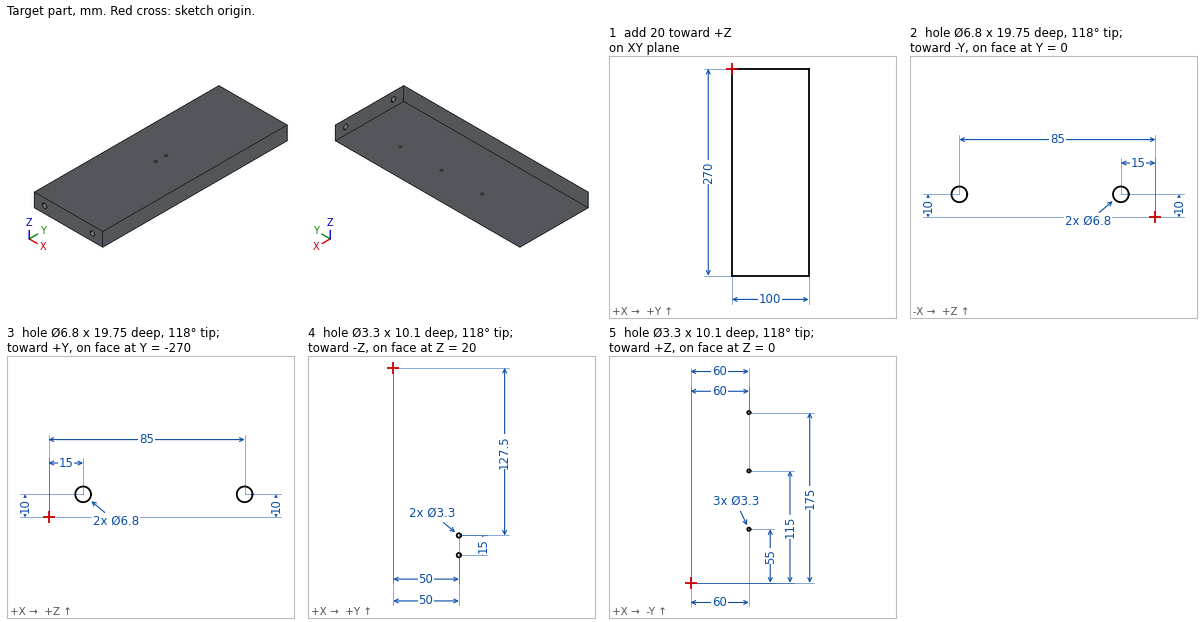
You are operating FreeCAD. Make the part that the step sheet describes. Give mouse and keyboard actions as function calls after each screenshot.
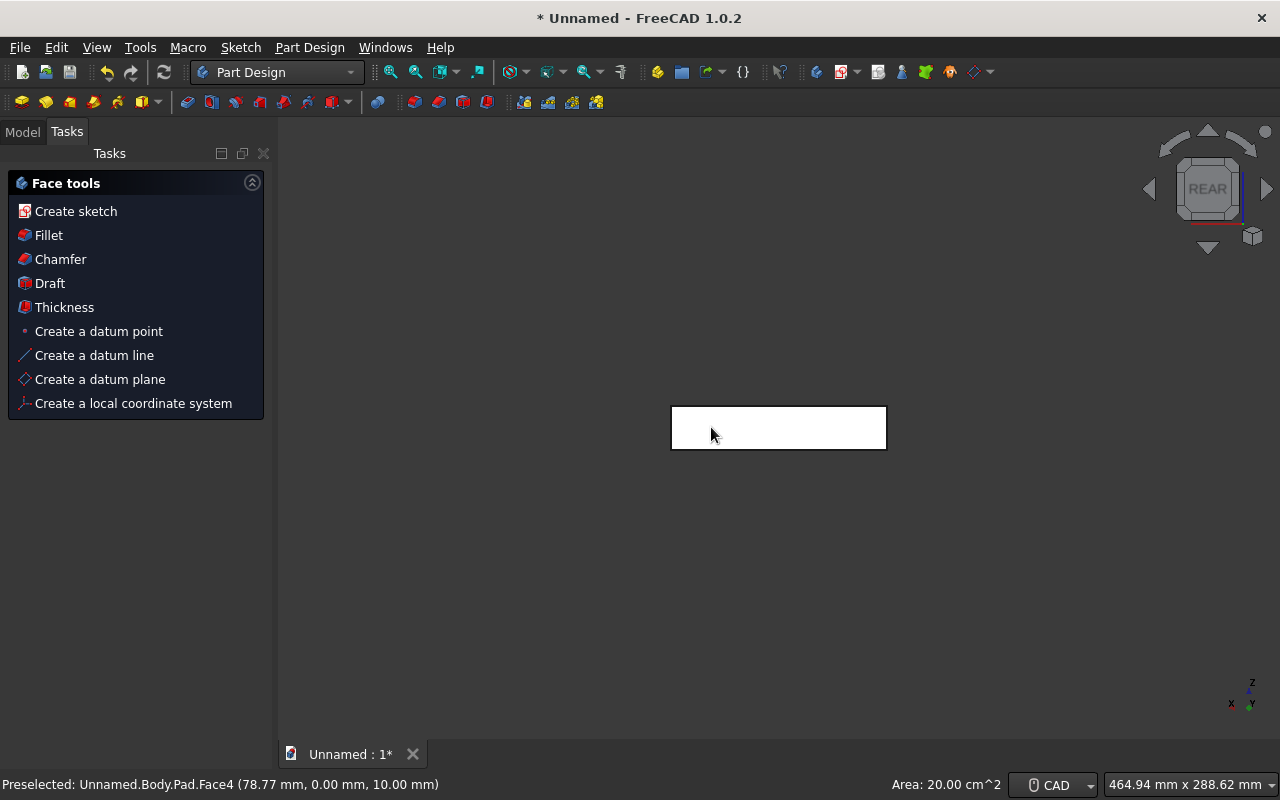
click(842, 72)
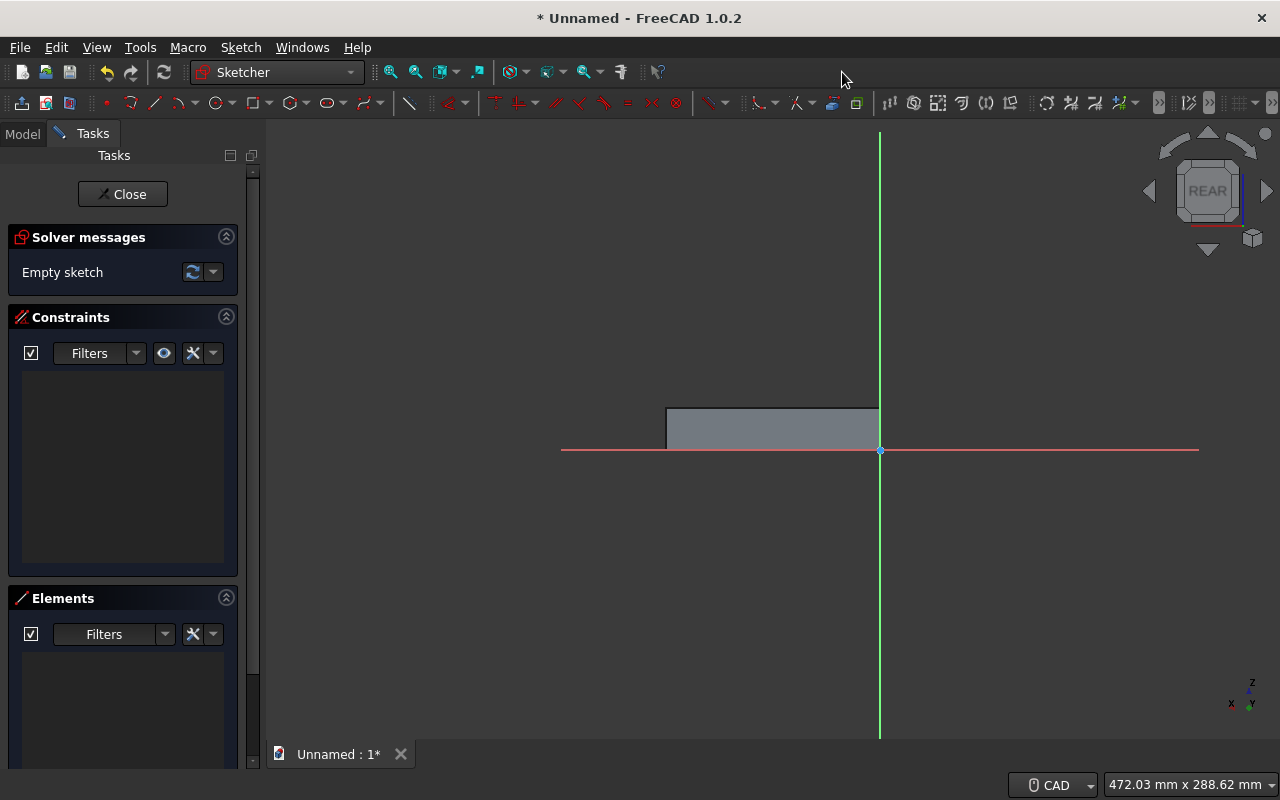
scroll(820, 439, up, 6)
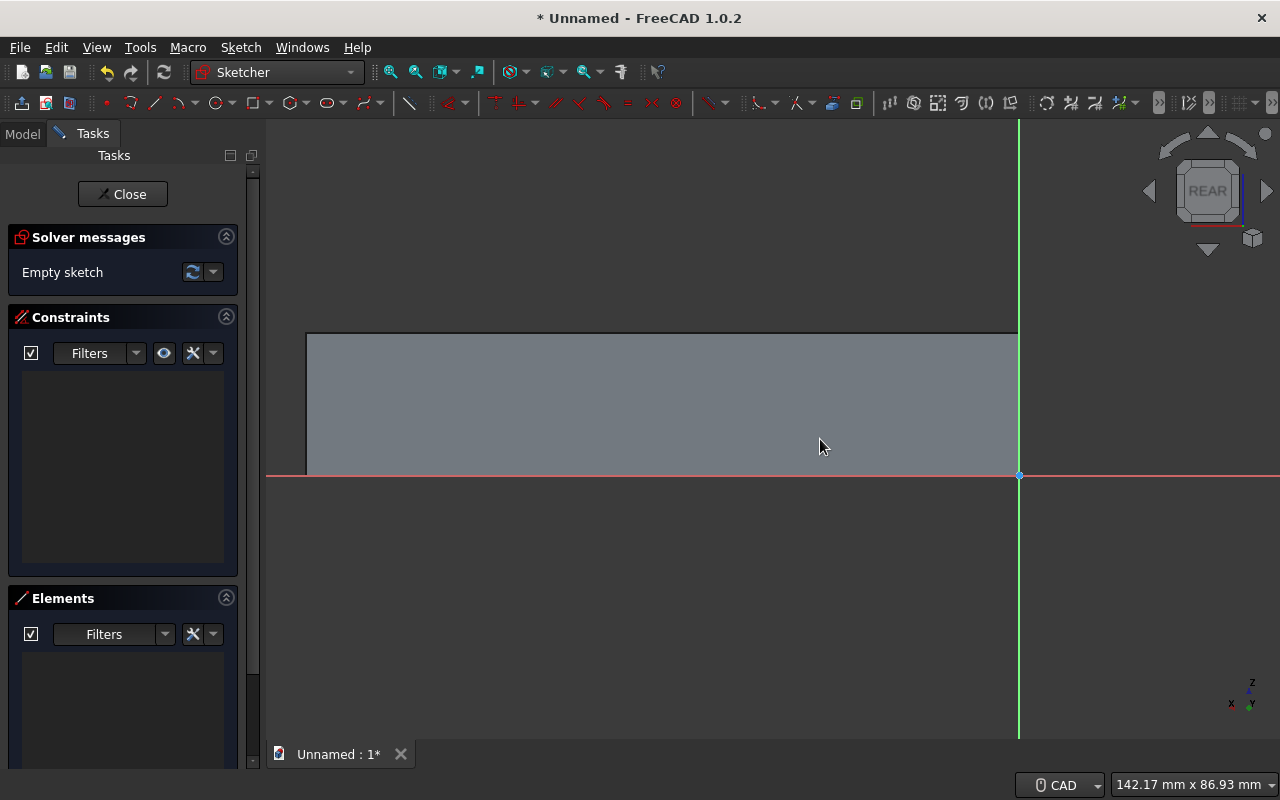
click(216, 104)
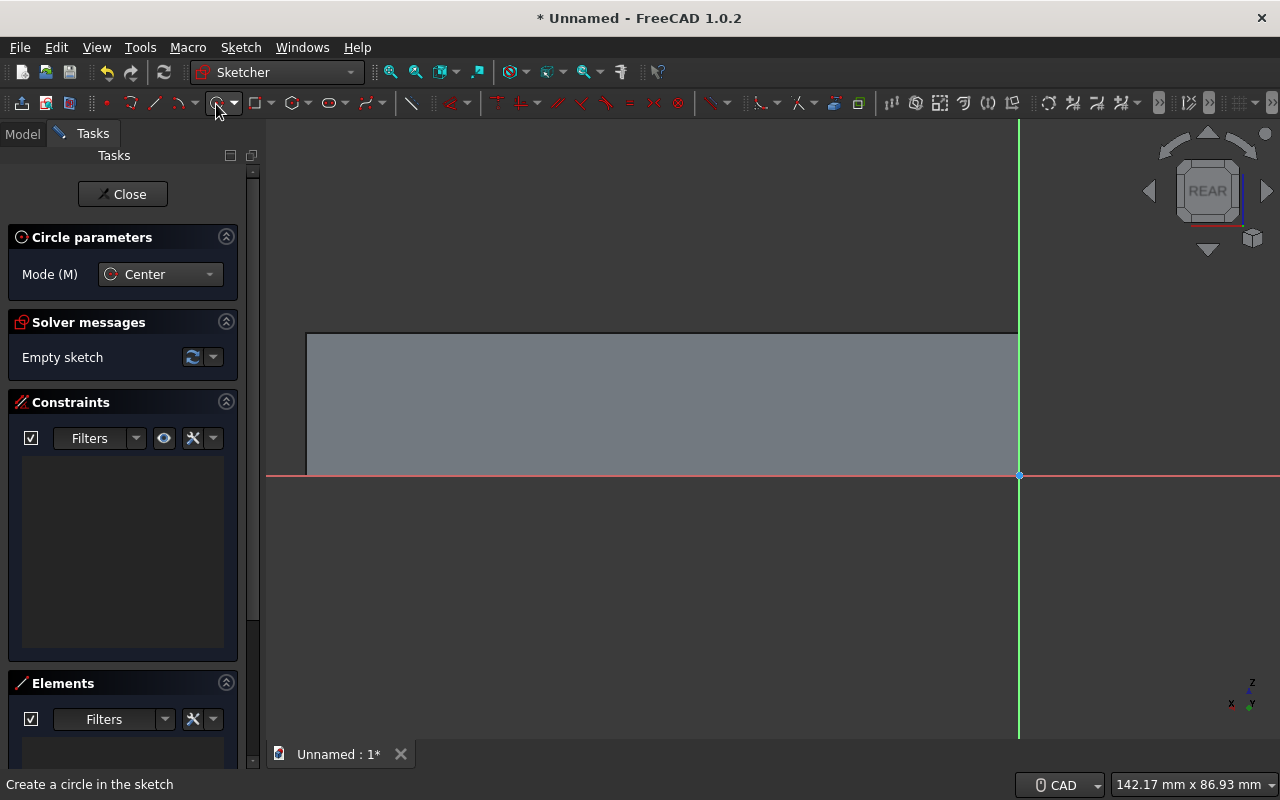
click(912, 405)
click(929, 387)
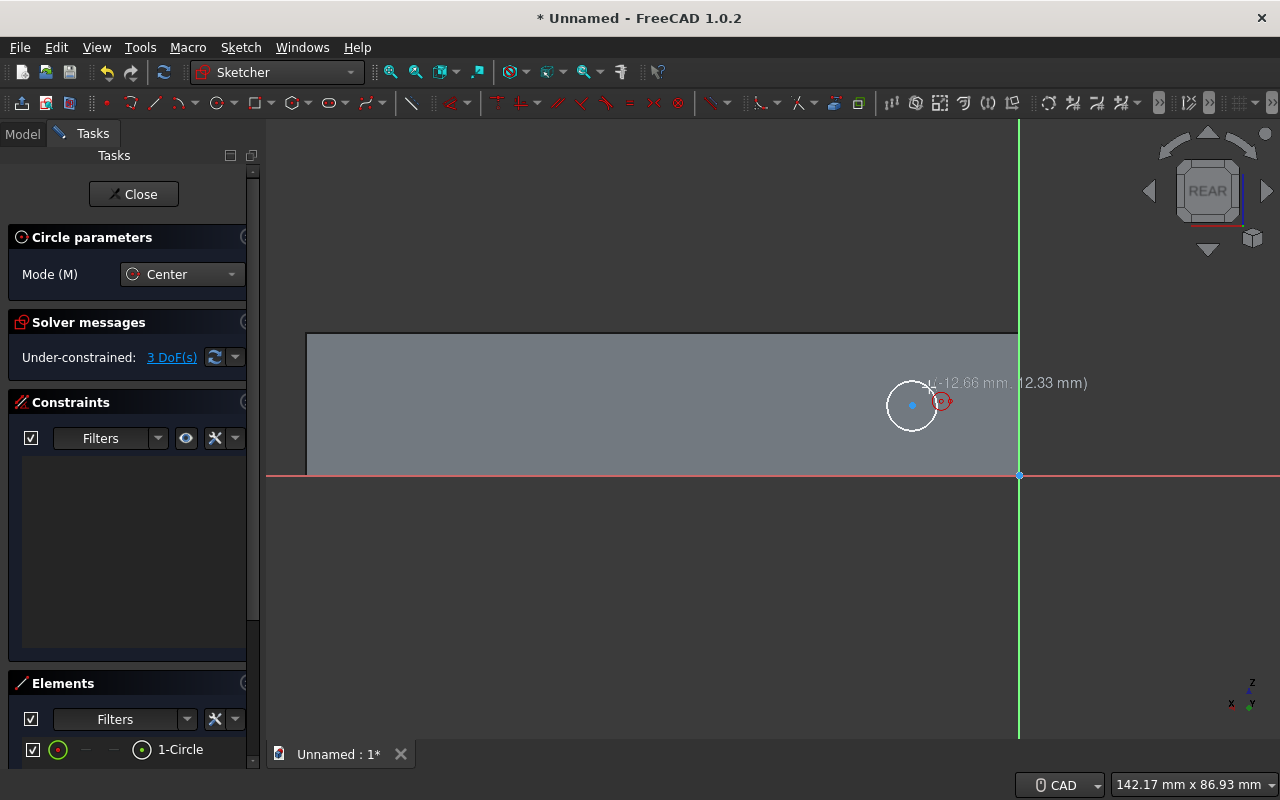
click(413, 405)
click(430, 387)
key(Escape)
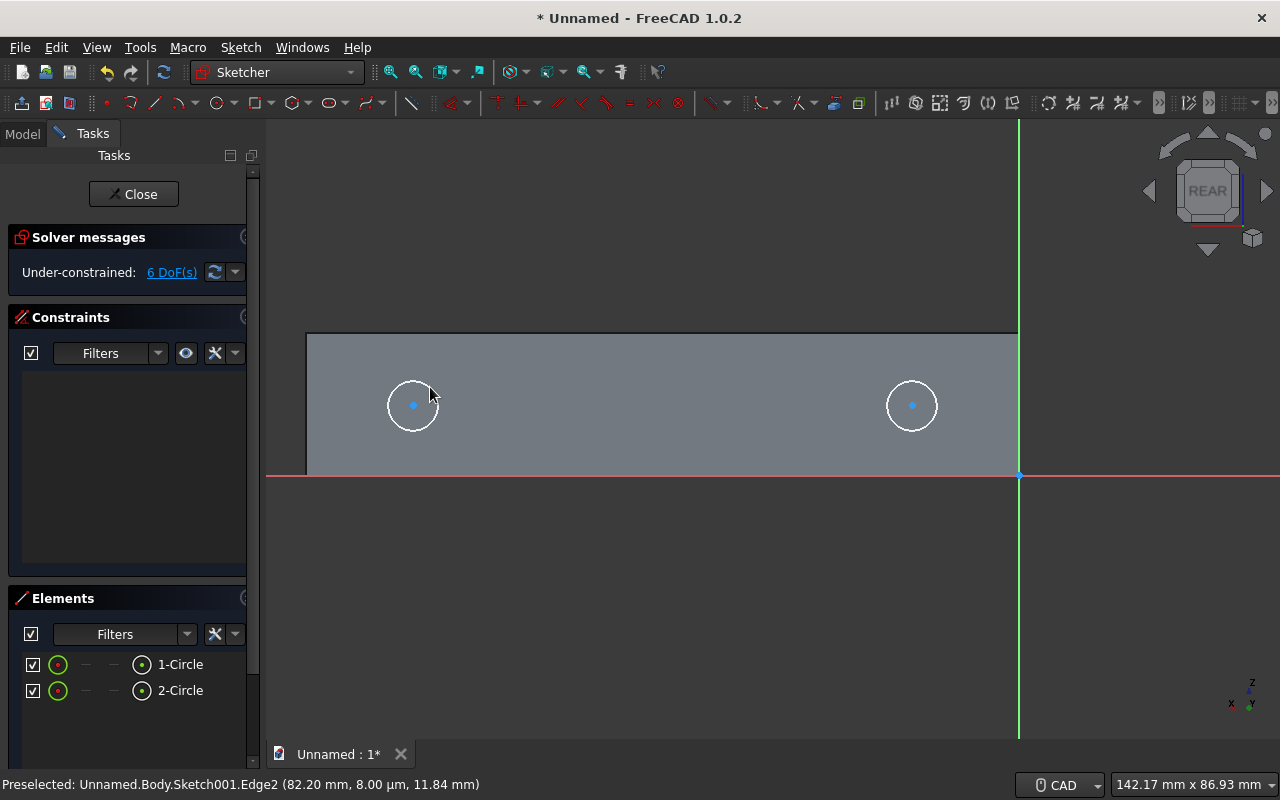
click(929, 388)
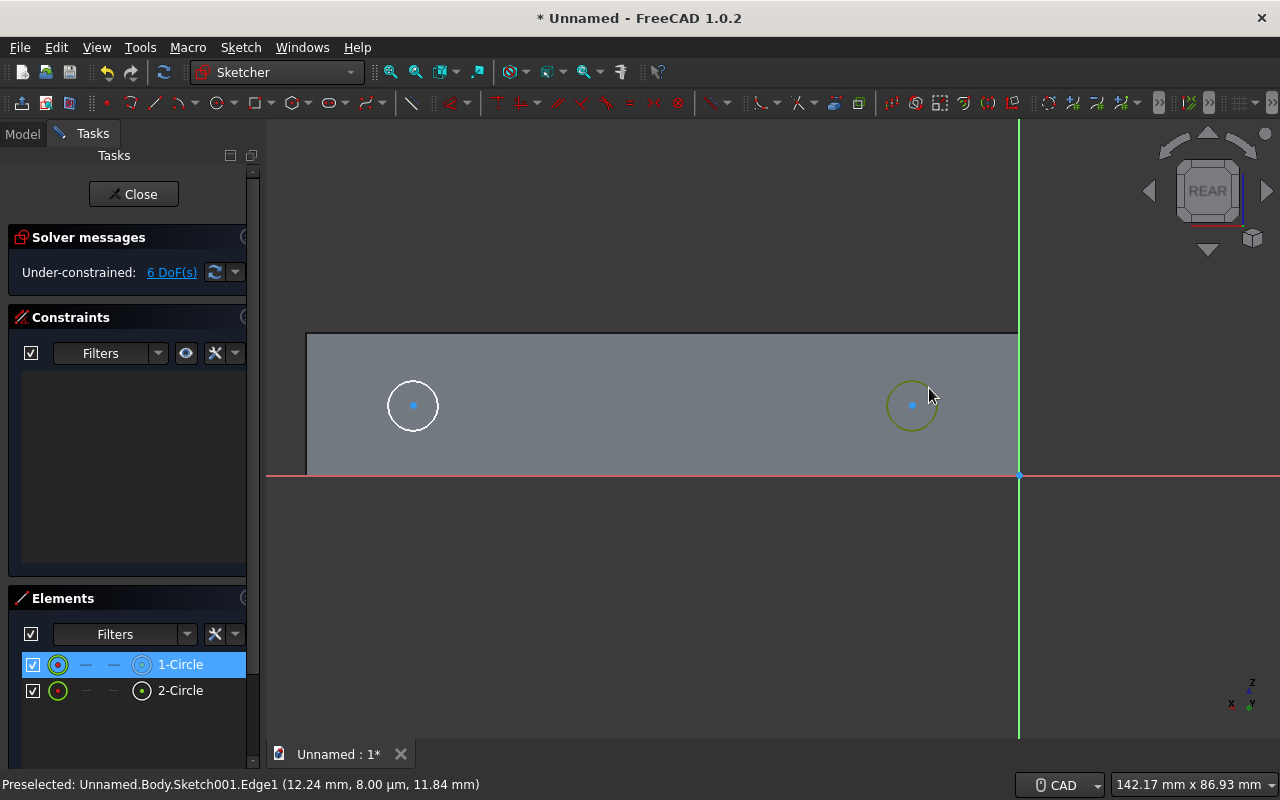
click(430, 388)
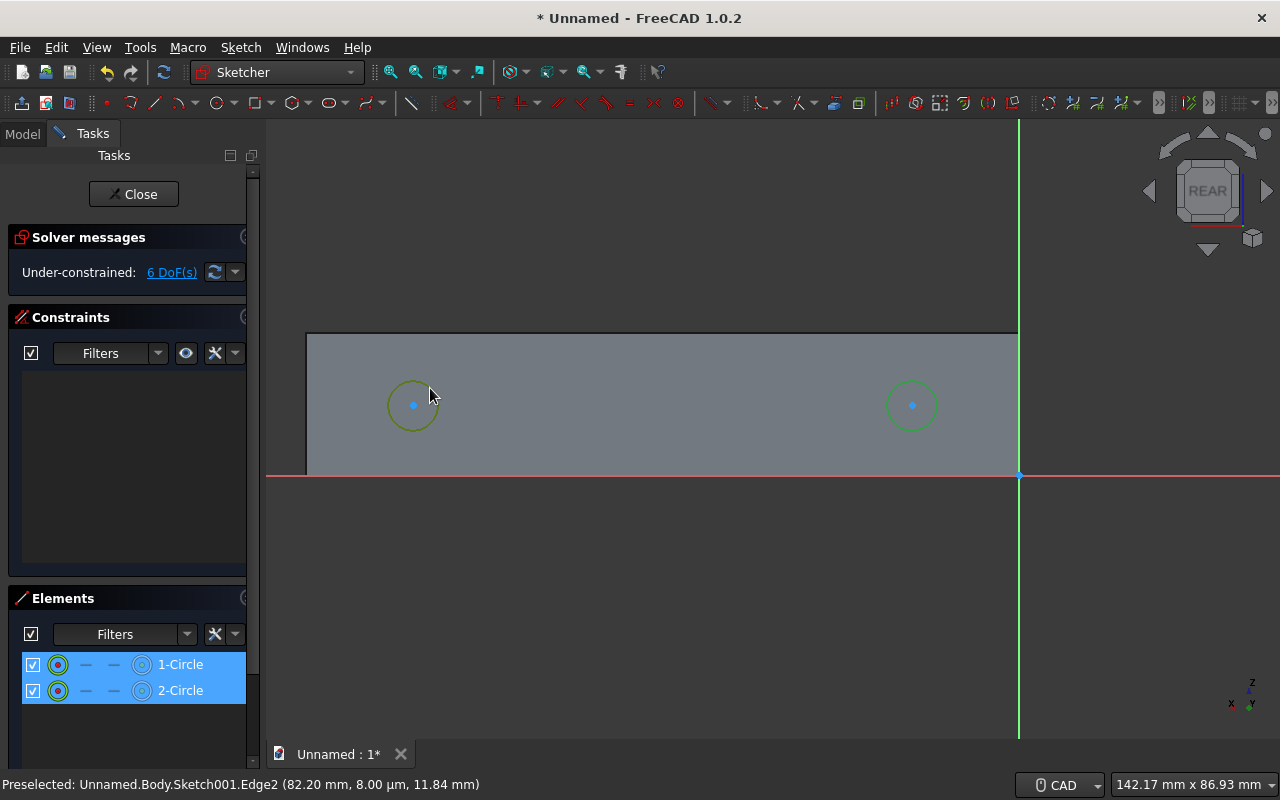
key(e)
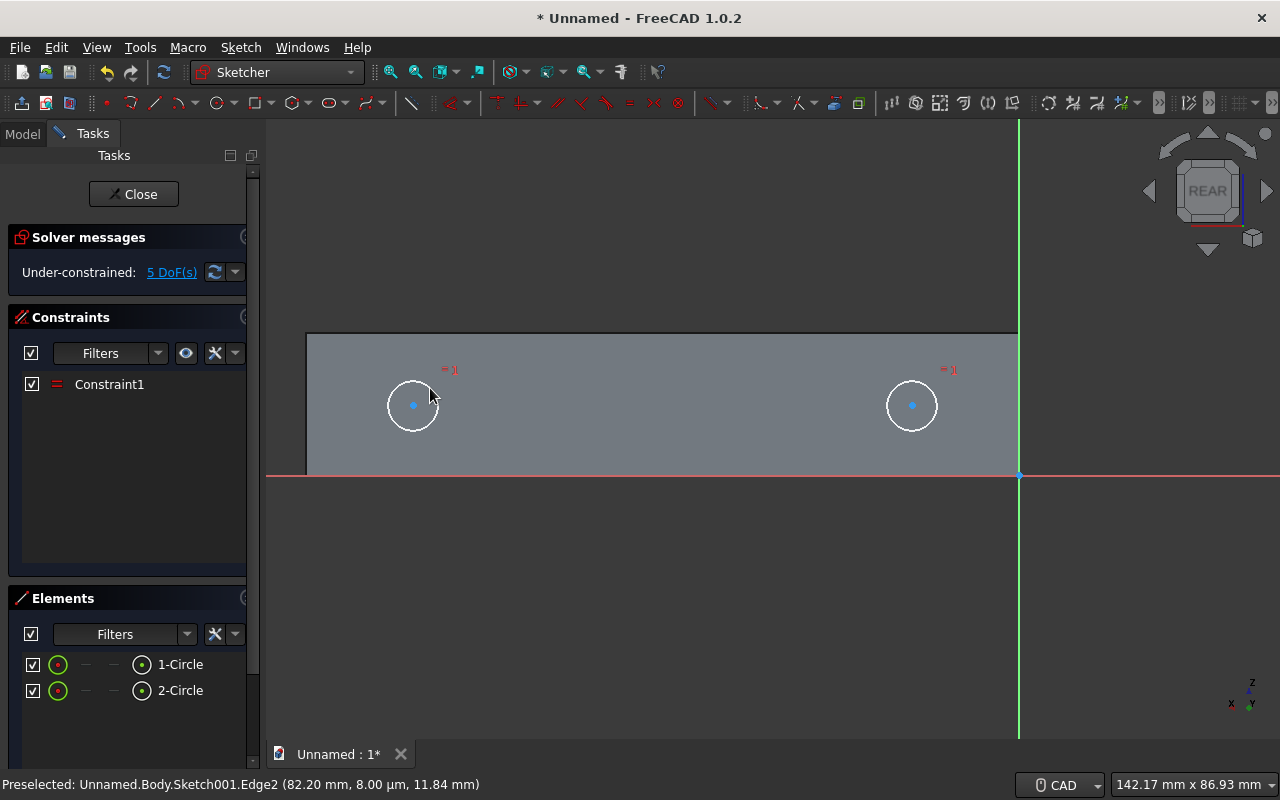
click(450, 104)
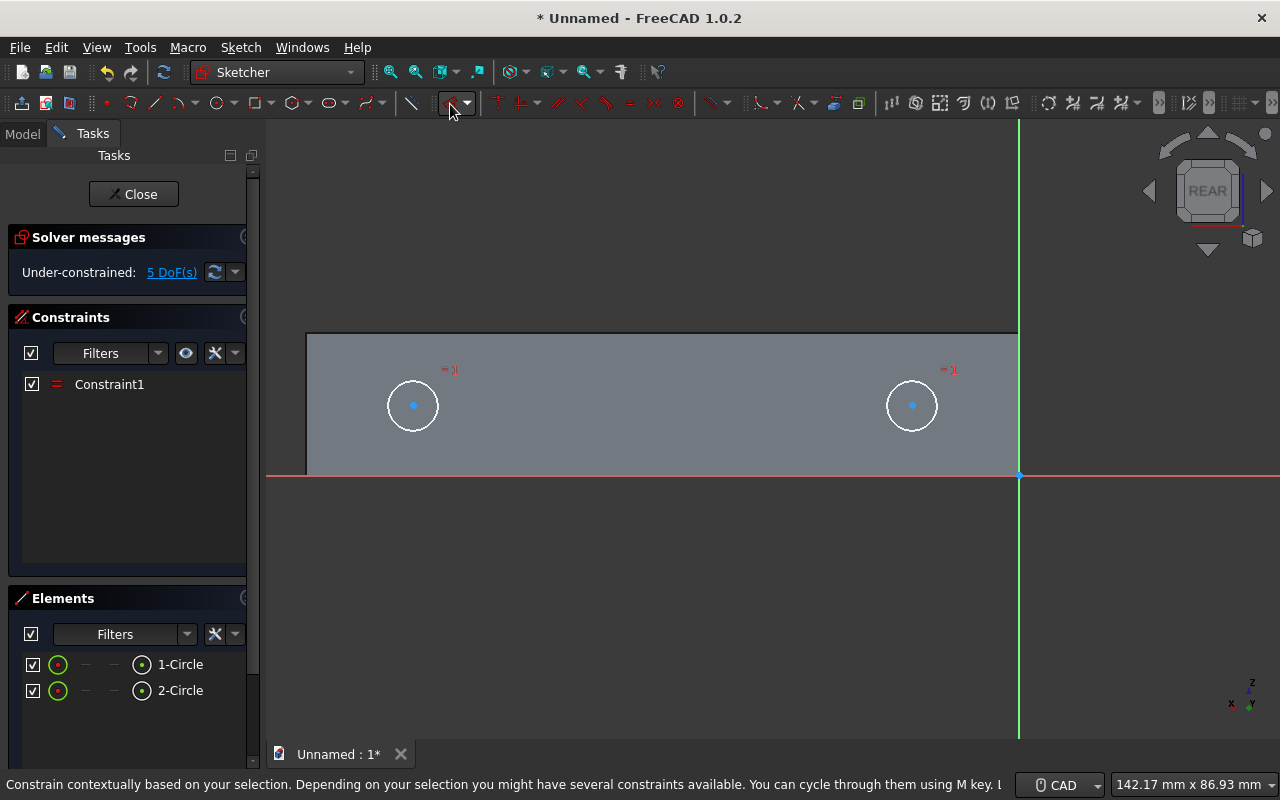
click(929, 388)
click(951, 365)